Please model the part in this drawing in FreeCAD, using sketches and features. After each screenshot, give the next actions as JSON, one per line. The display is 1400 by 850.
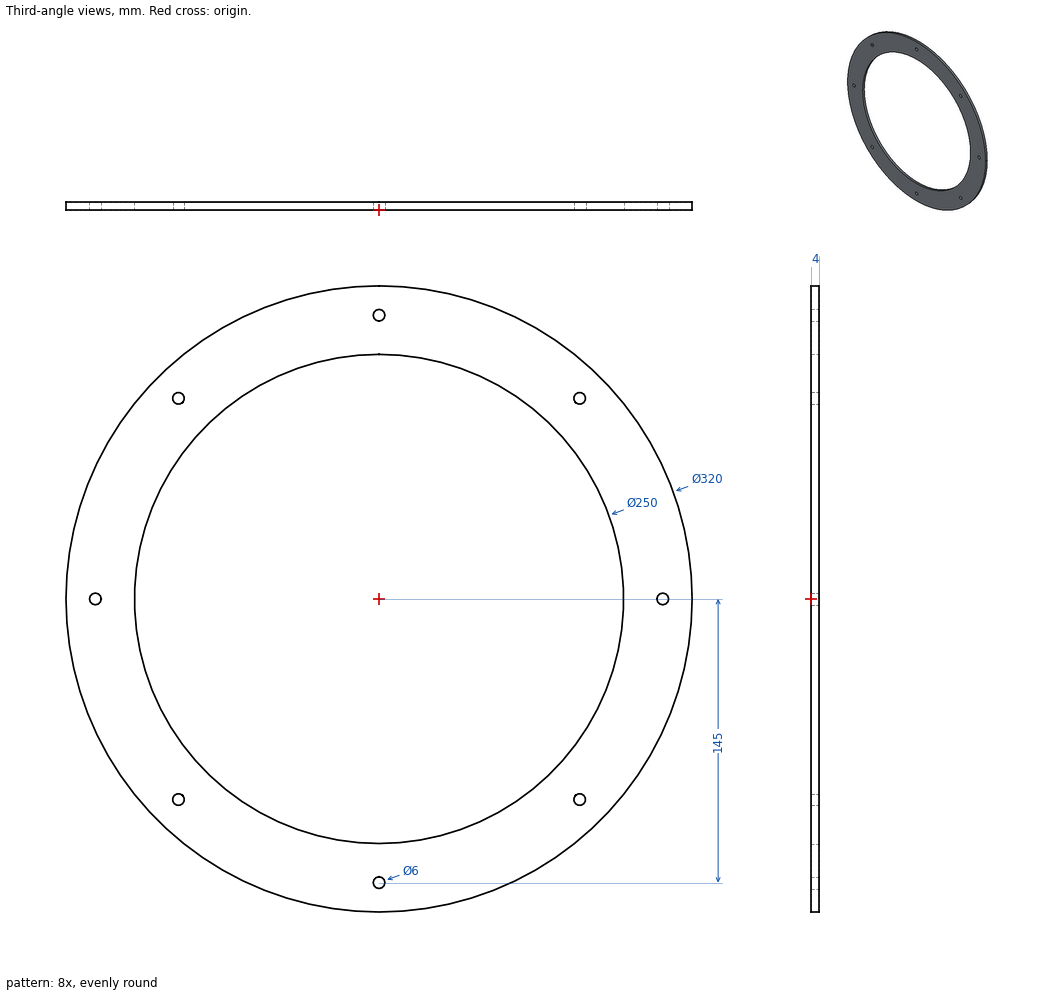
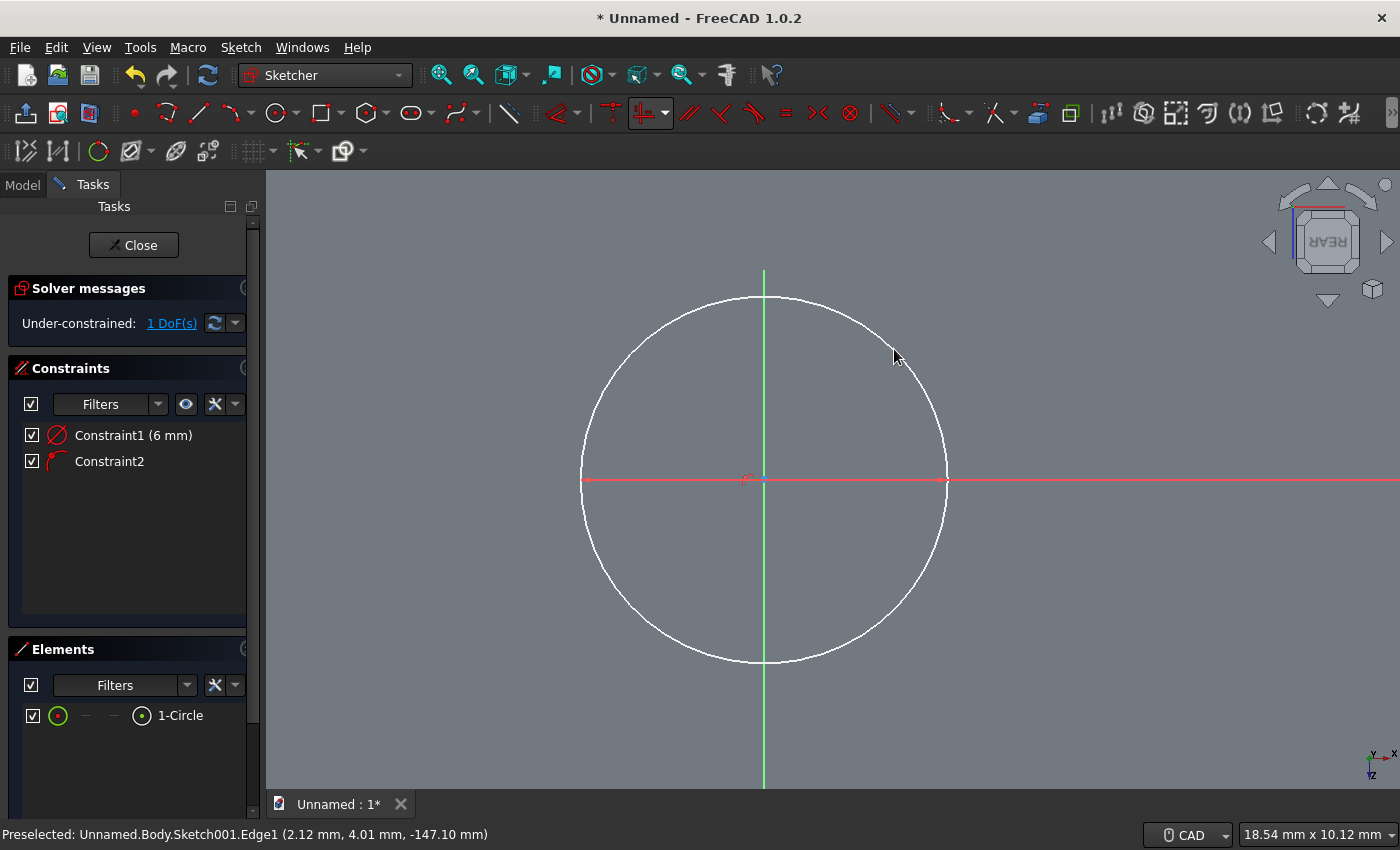
{"action": "key", "text": "d"}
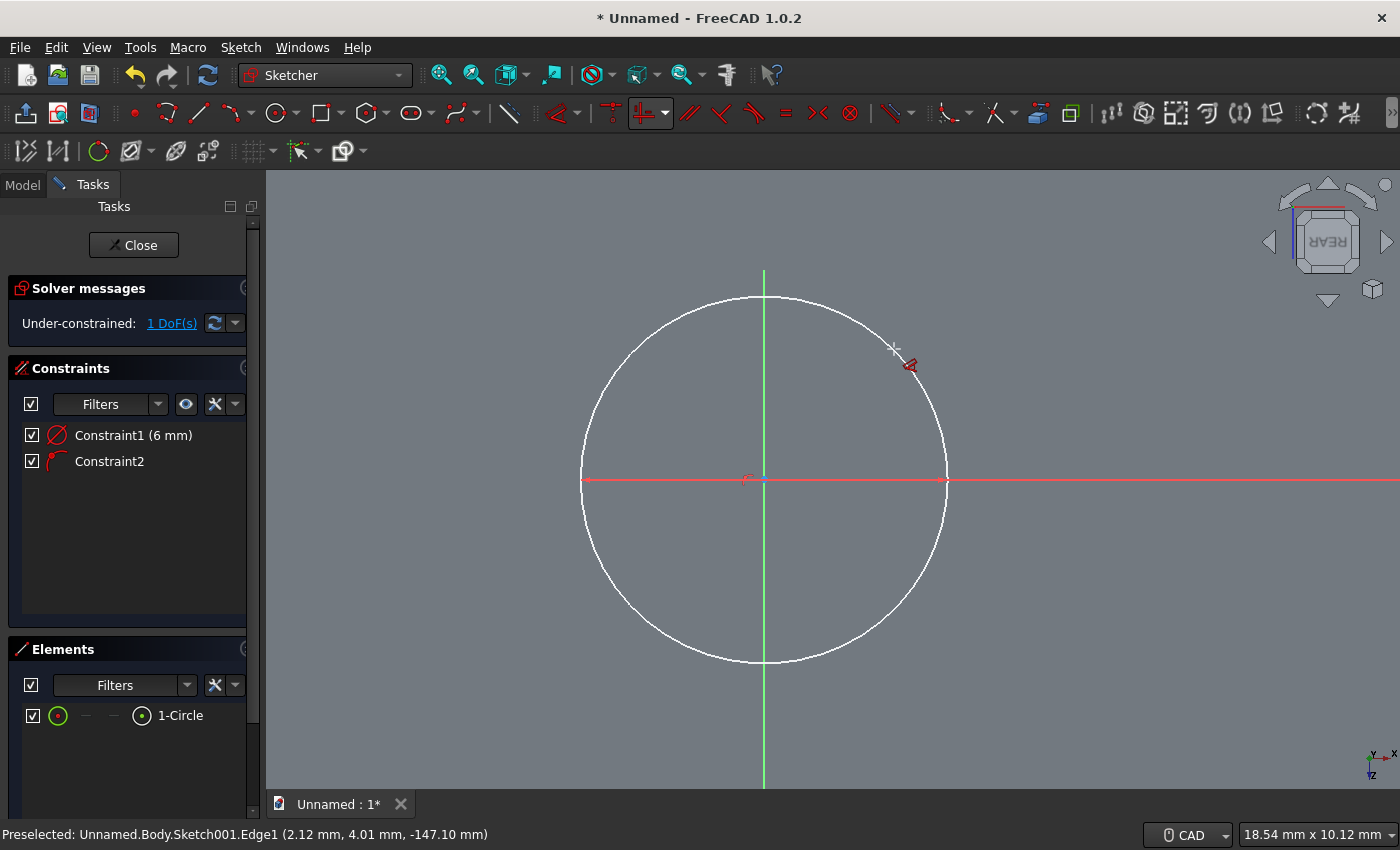
{"action": "left_click", "coordinate": [764, 480]}
{"action": "left_click", "coordinate": [798, 621]}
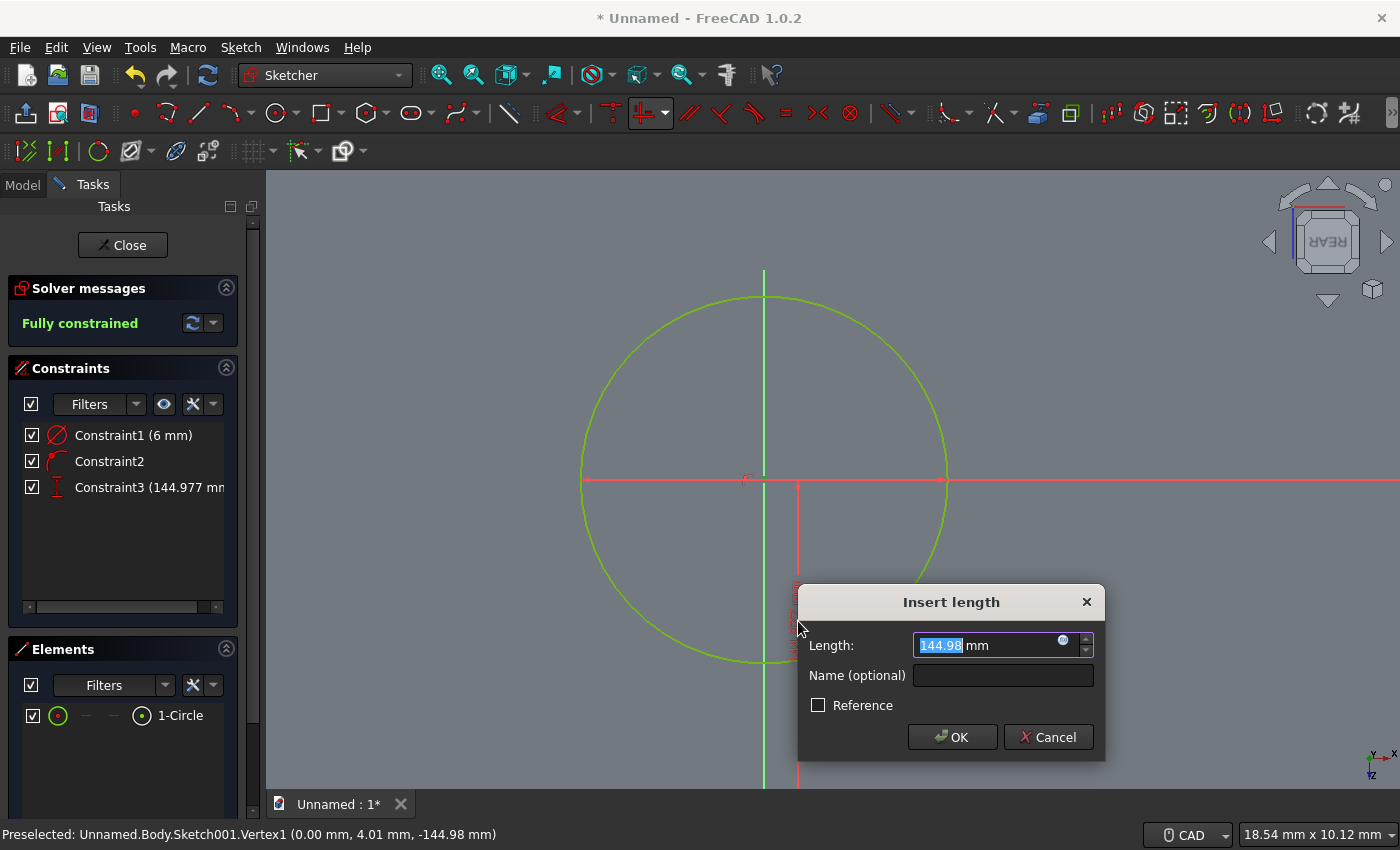
{"action": "type", "text": "145"}
{"action": "key", "text": "Return"}
{"action": "key", "text": "Escape"}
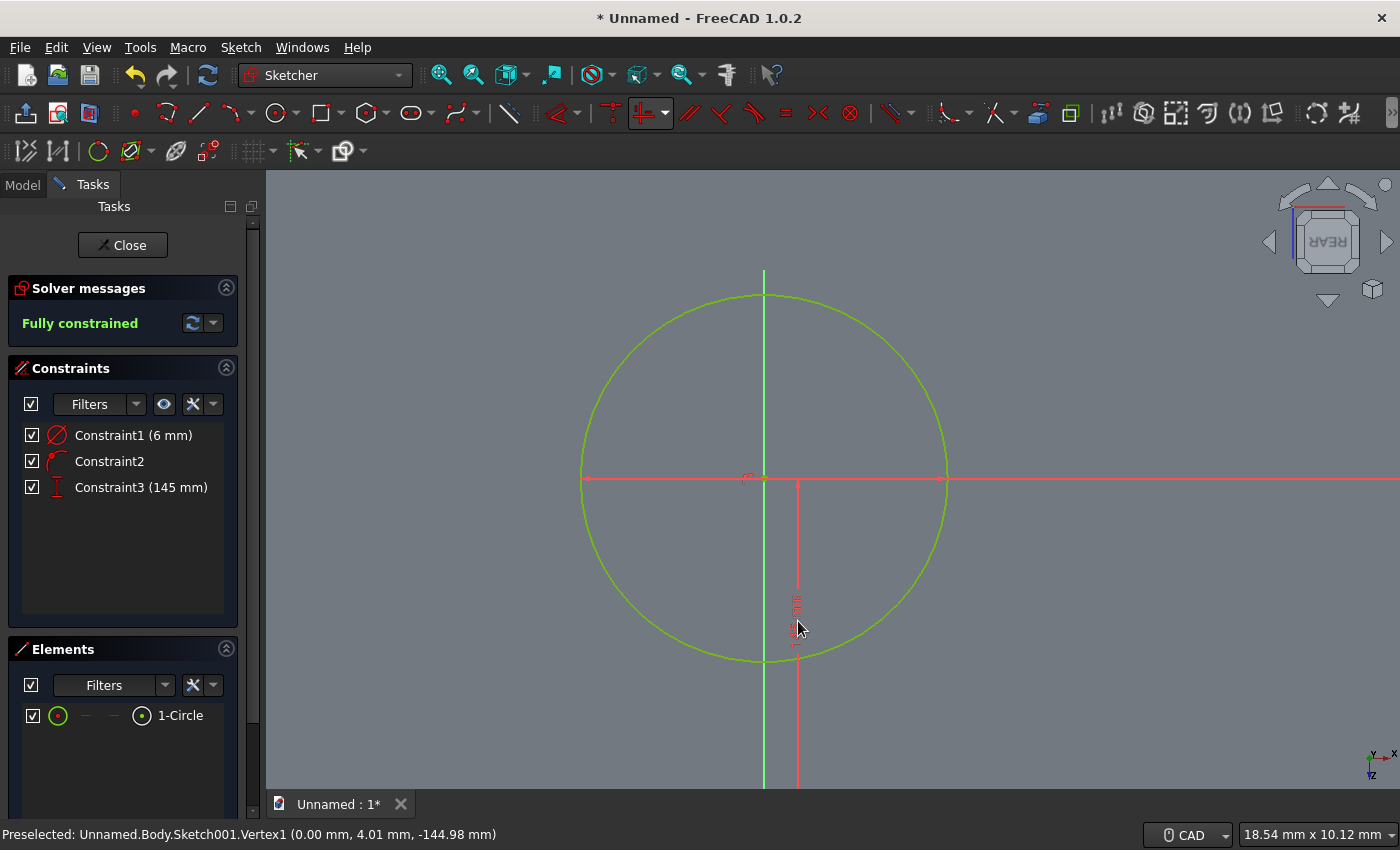
{"action": "left_click", "coordinate": [123, 245]}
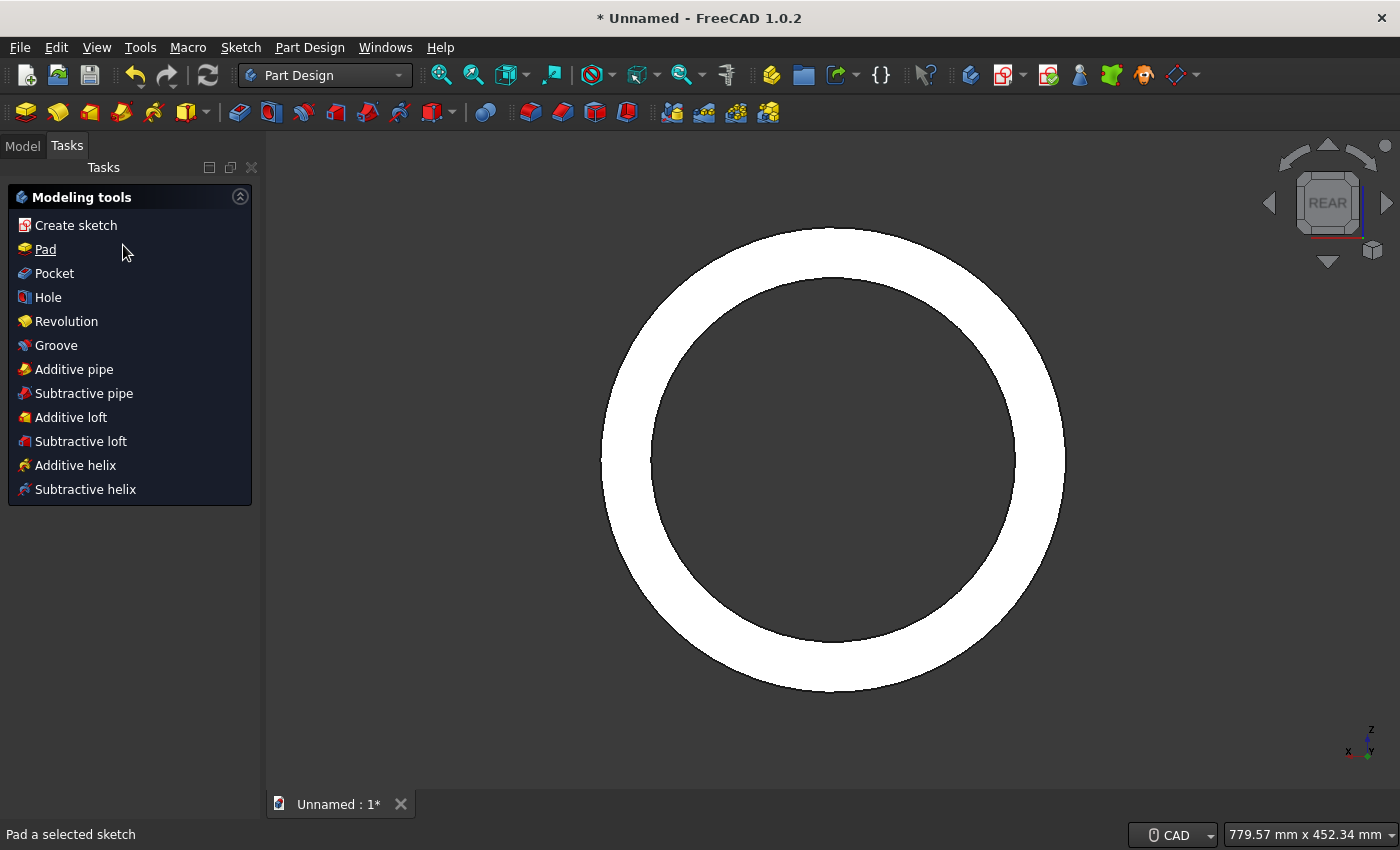
{"action": "left_click", "coordinate": [240, 112]}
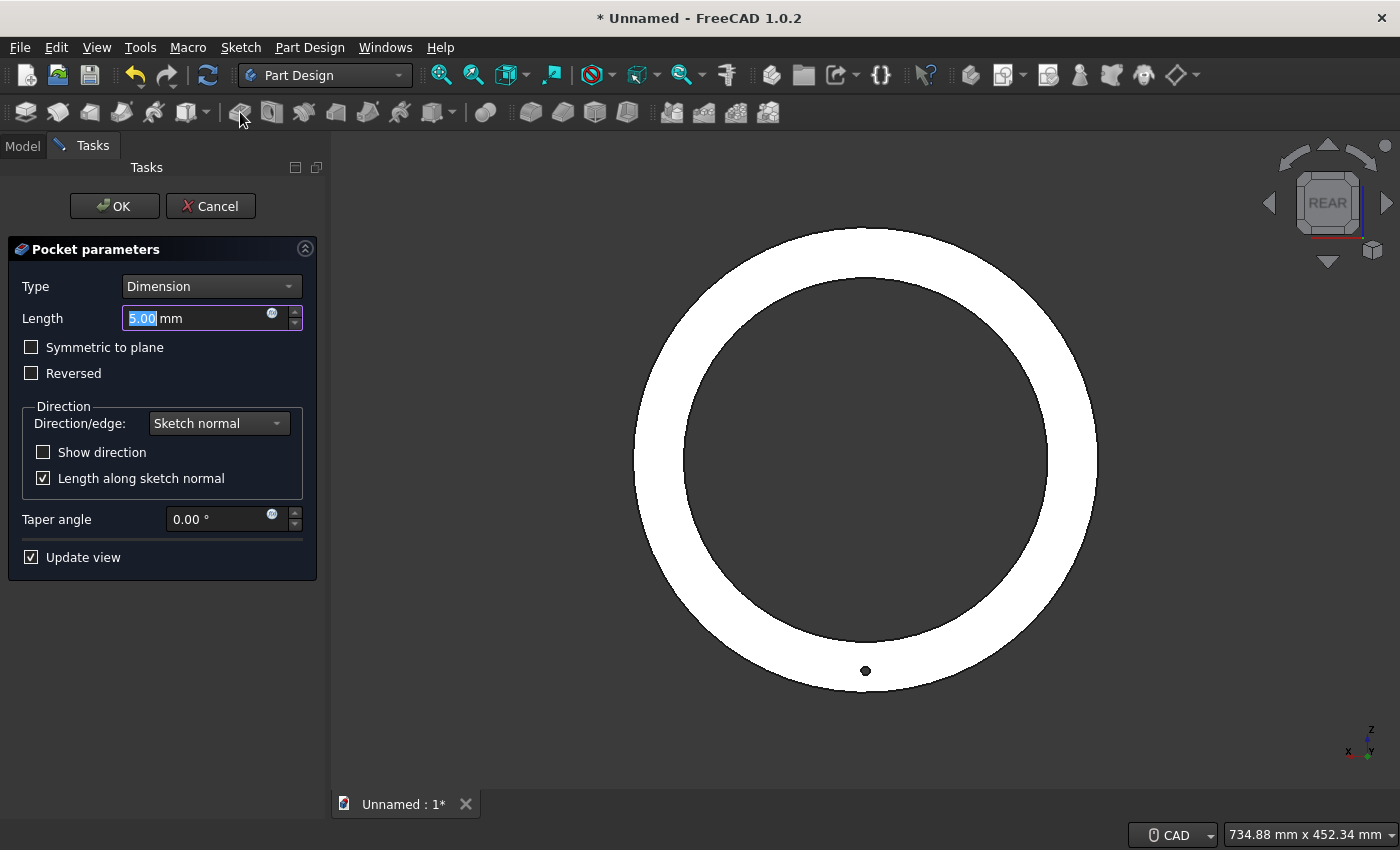
{"action": "left_click", "coordinate": [212, 286]}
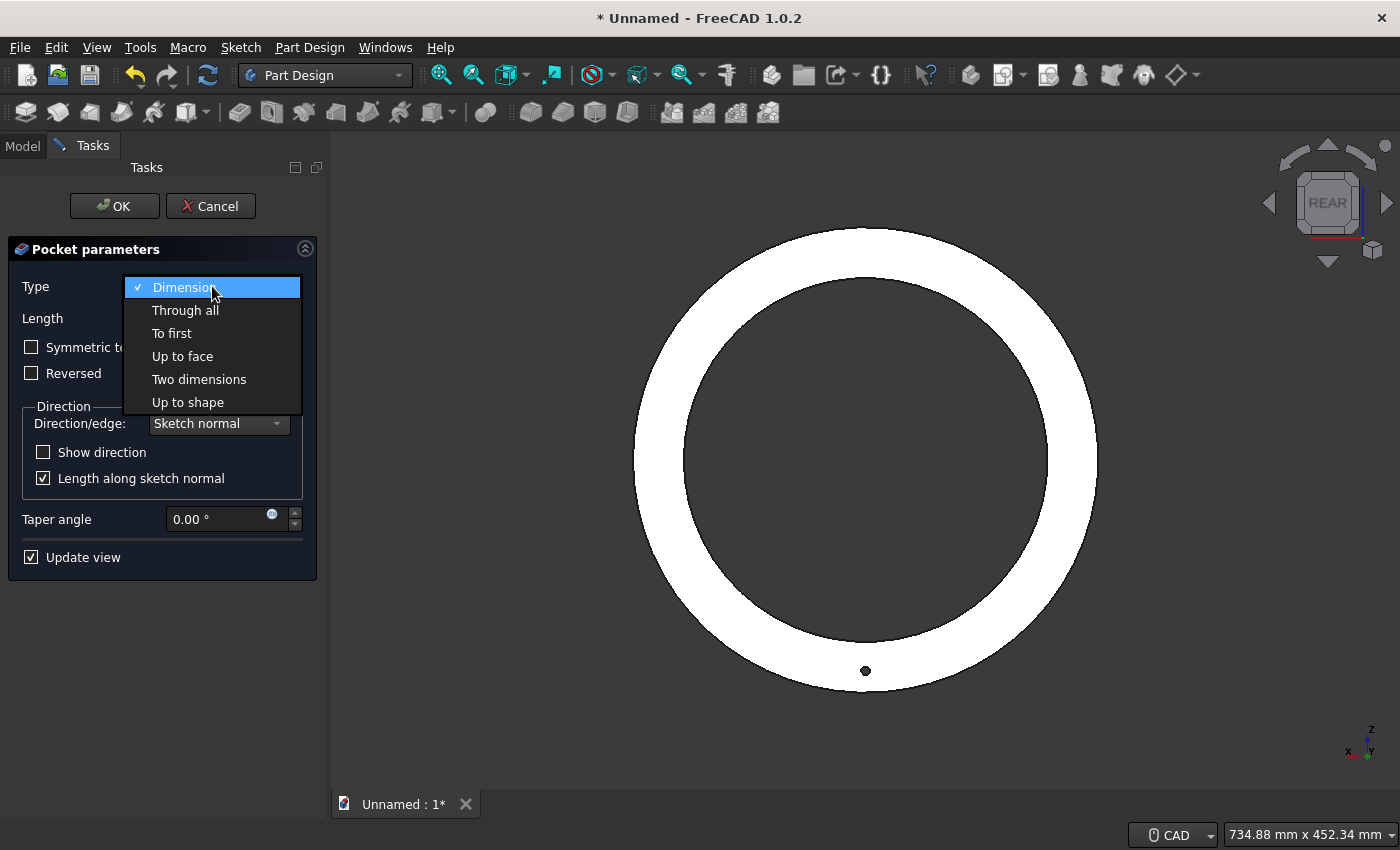
{"action": "left_click", "coordinate": [212, 310]}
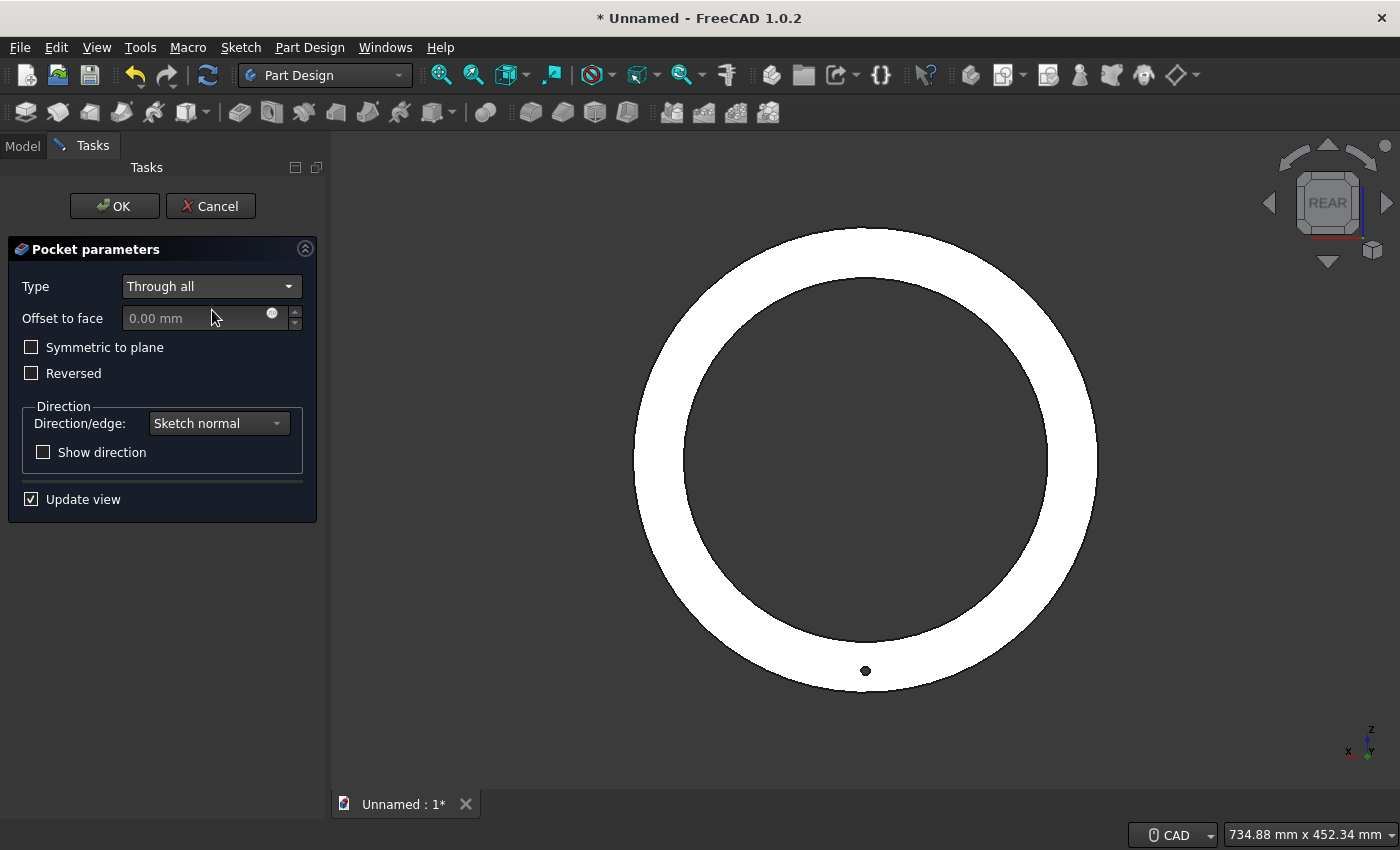
{"action": "left_click", "coordinate": [115, 206]}